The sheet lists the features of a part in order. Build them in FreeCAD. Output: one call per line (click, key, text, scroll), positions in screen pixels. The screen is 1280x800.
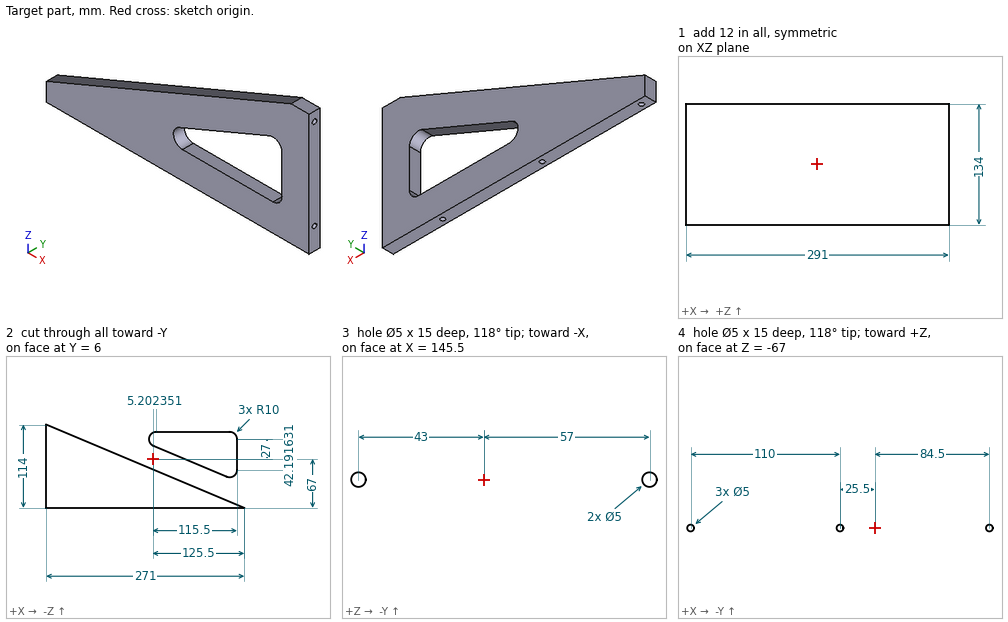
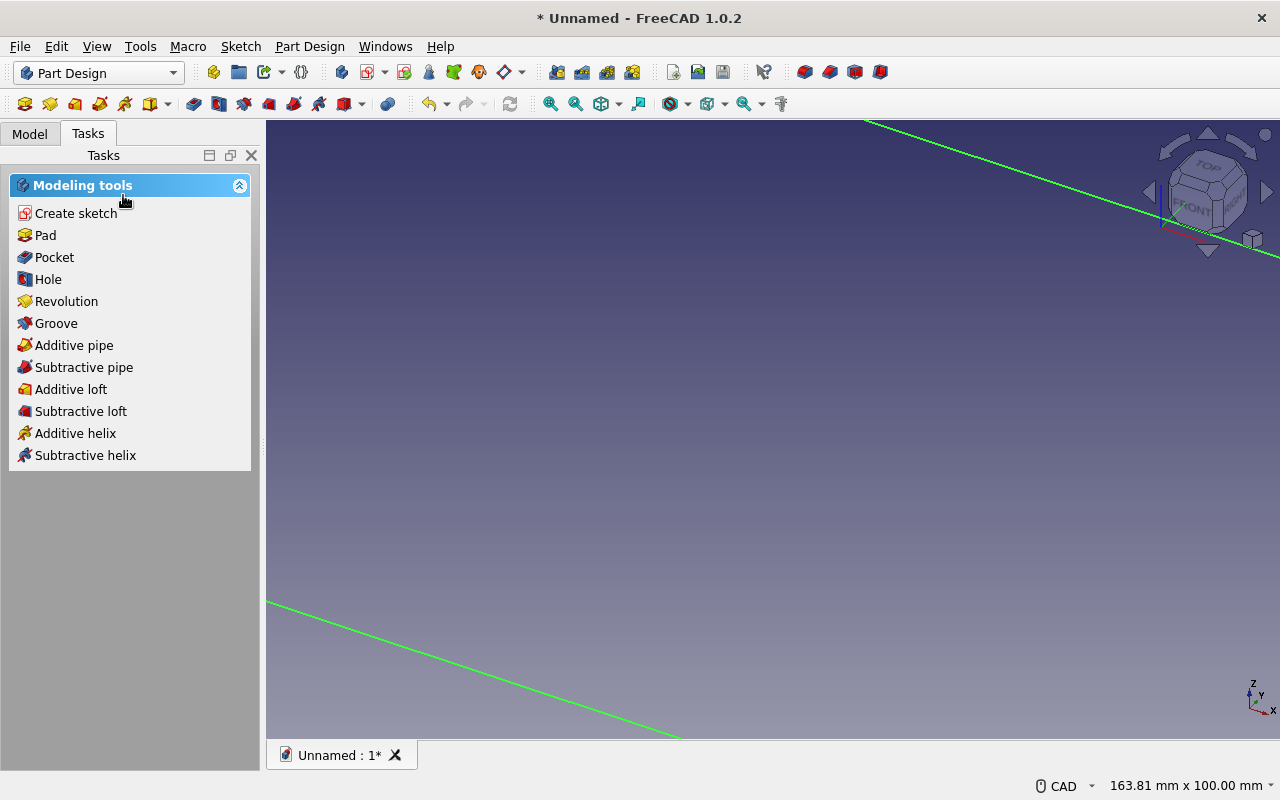
click(25, 104)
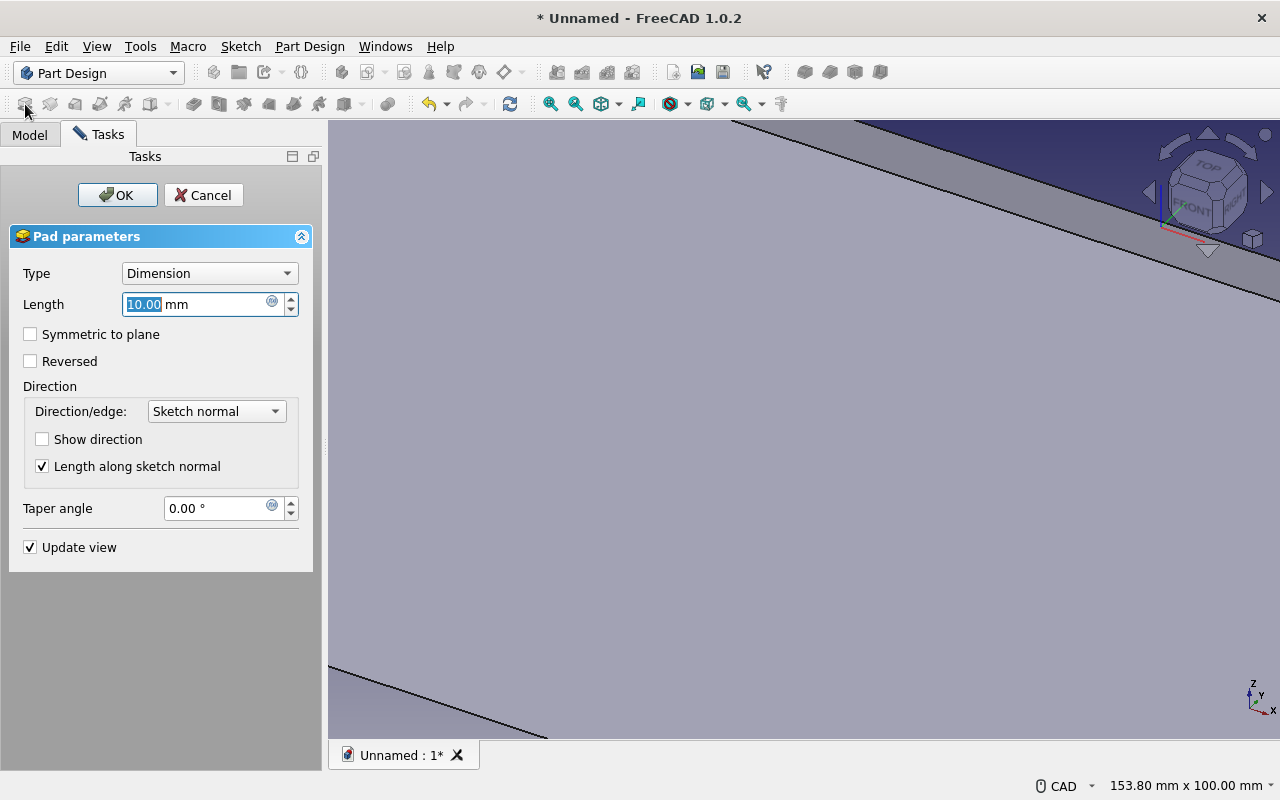
text(12)
key(Tab)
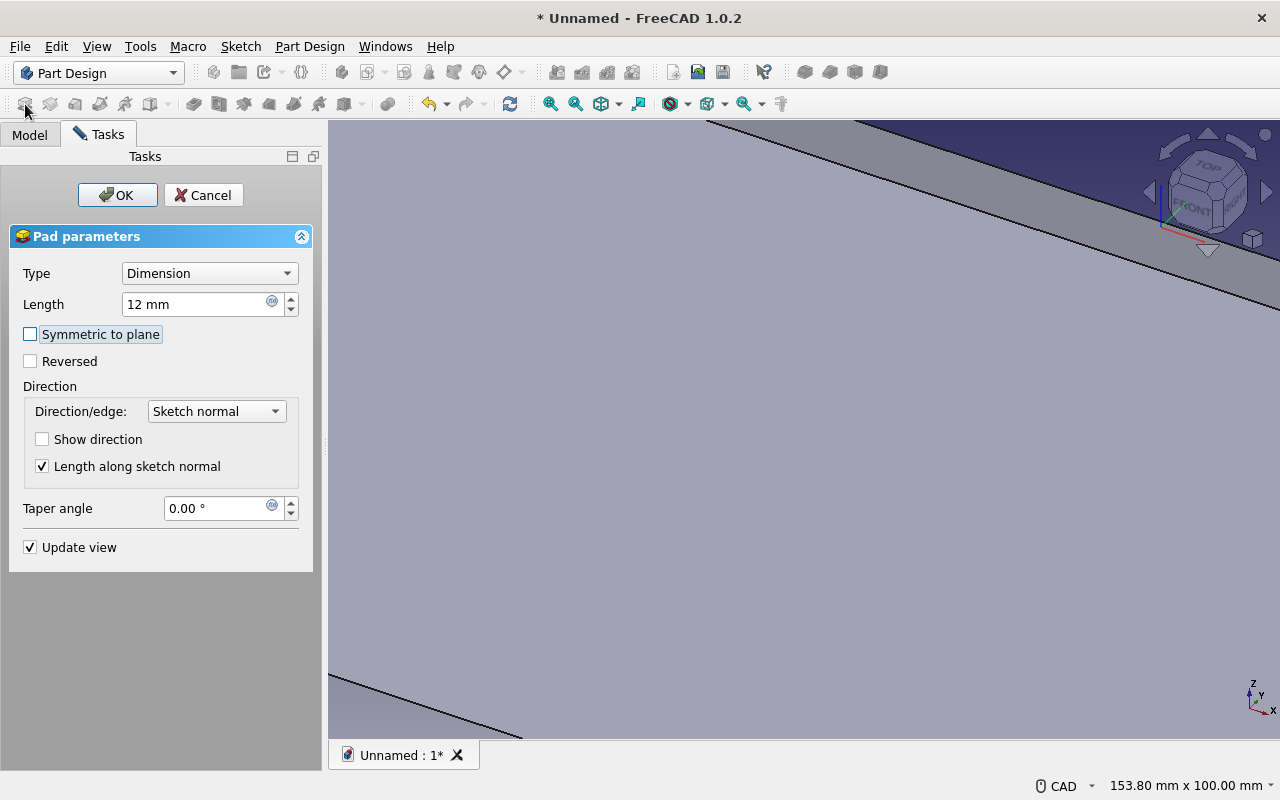
click(31, 334)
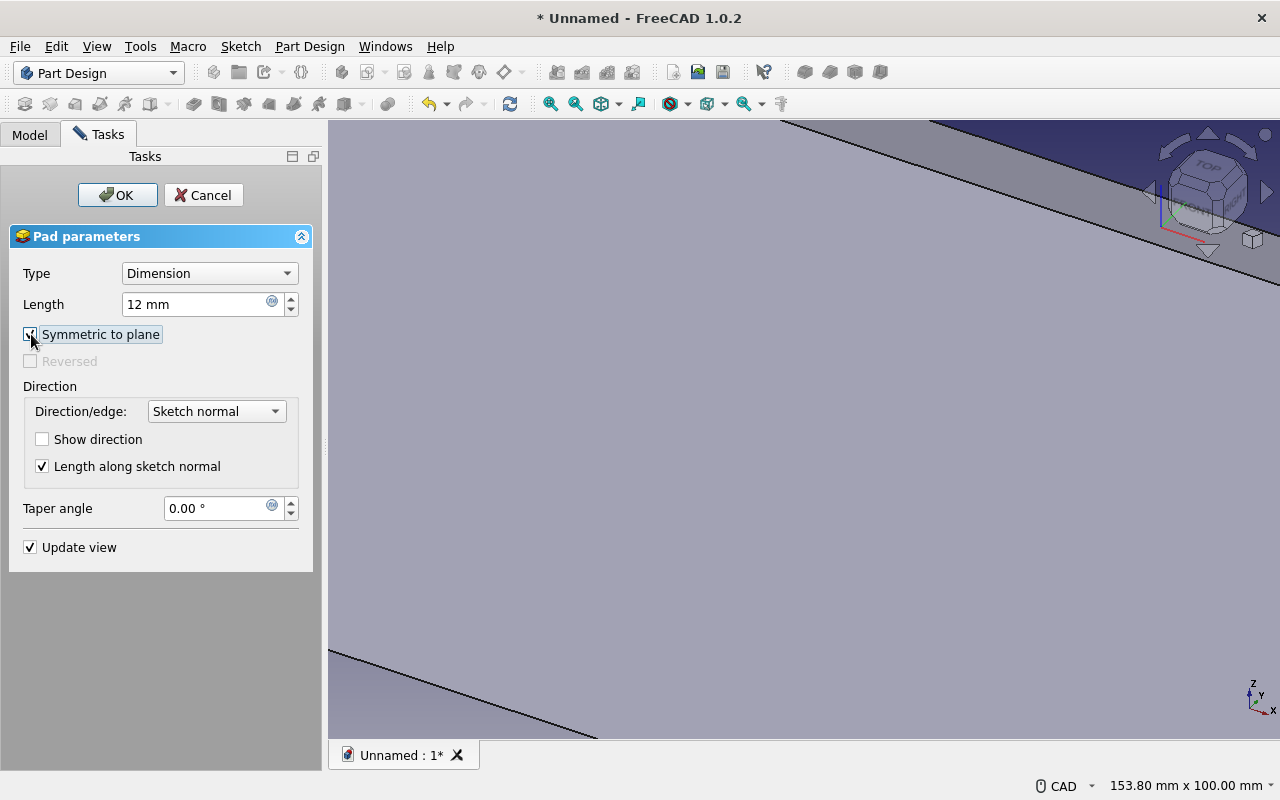
click(118, 195)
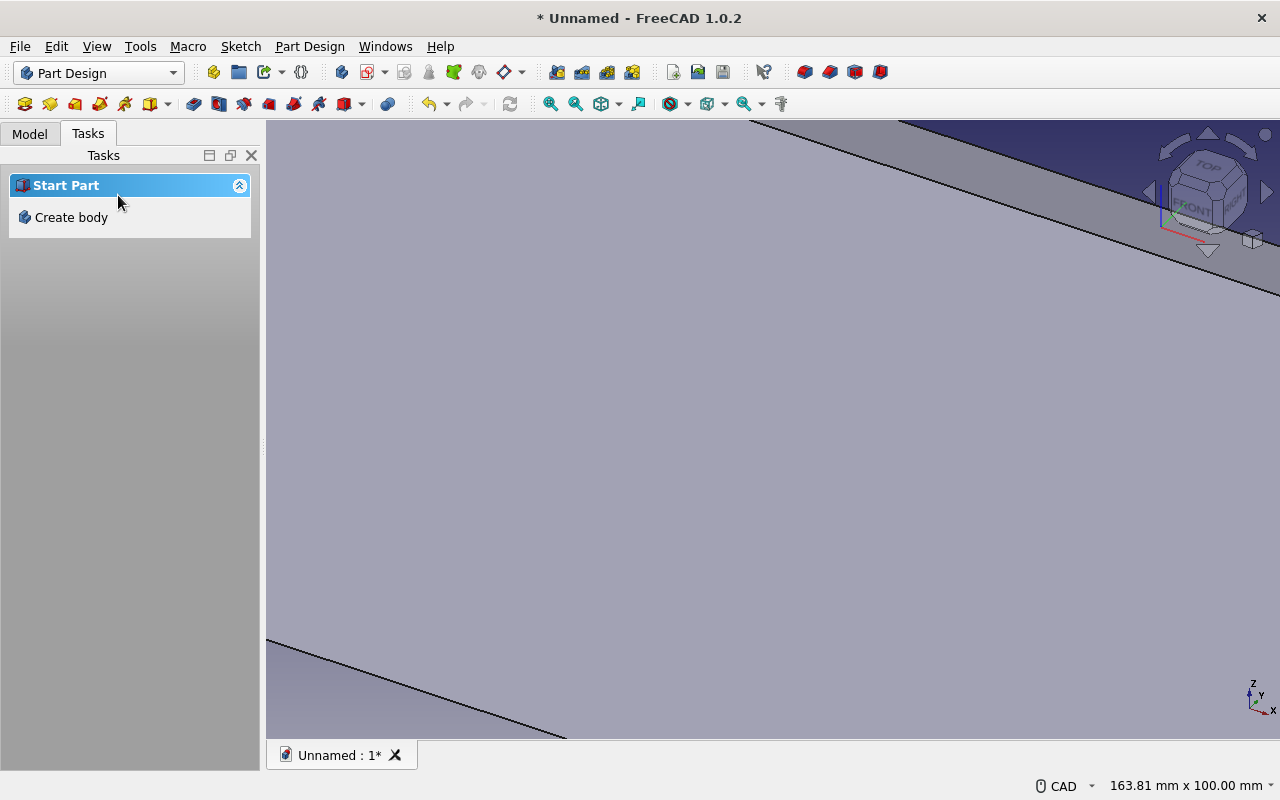
click(551, 104)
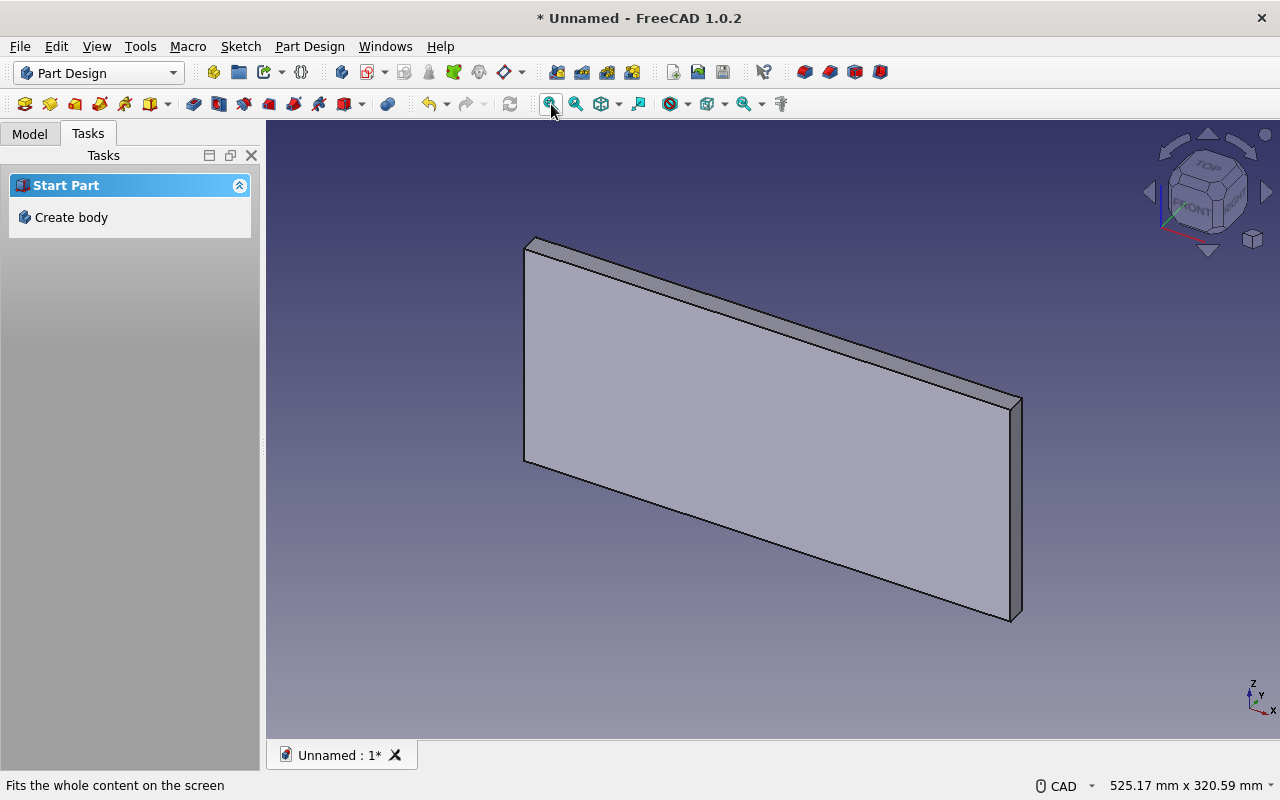
key(4)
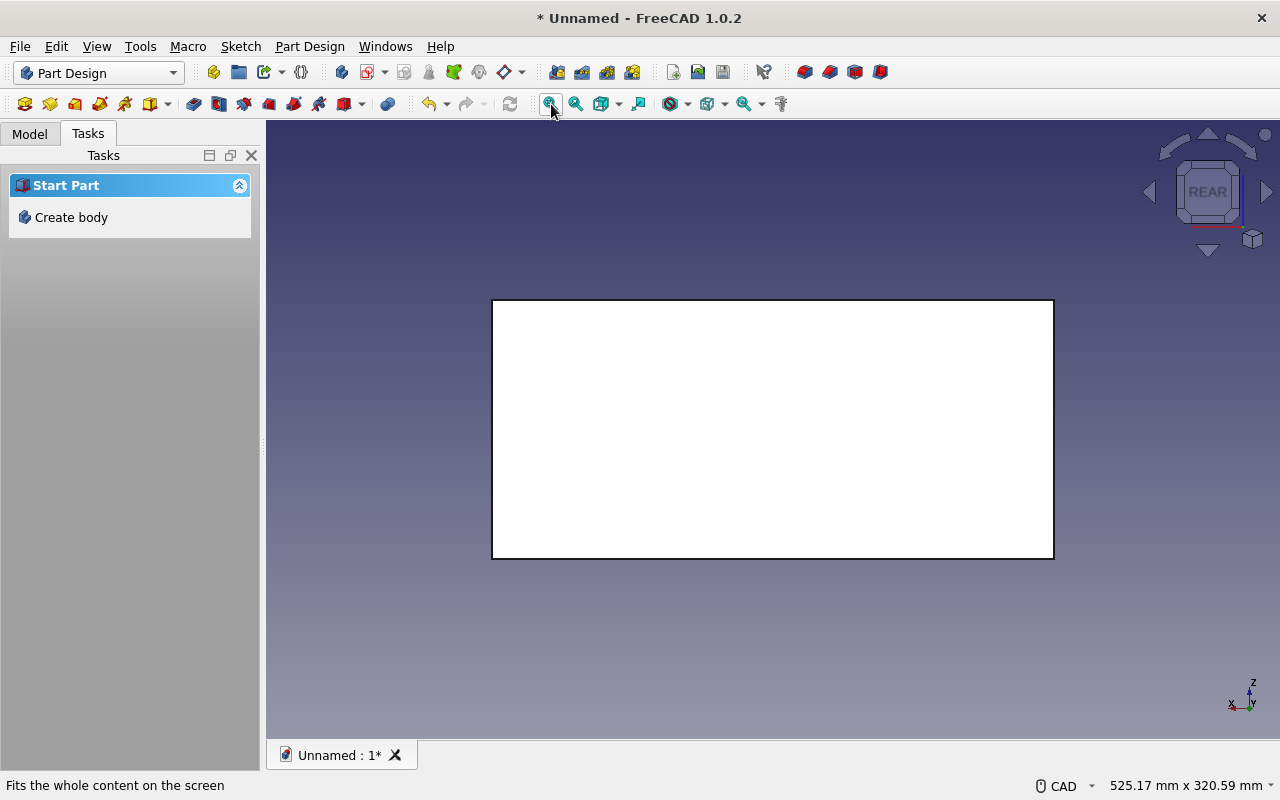
click(693, 429)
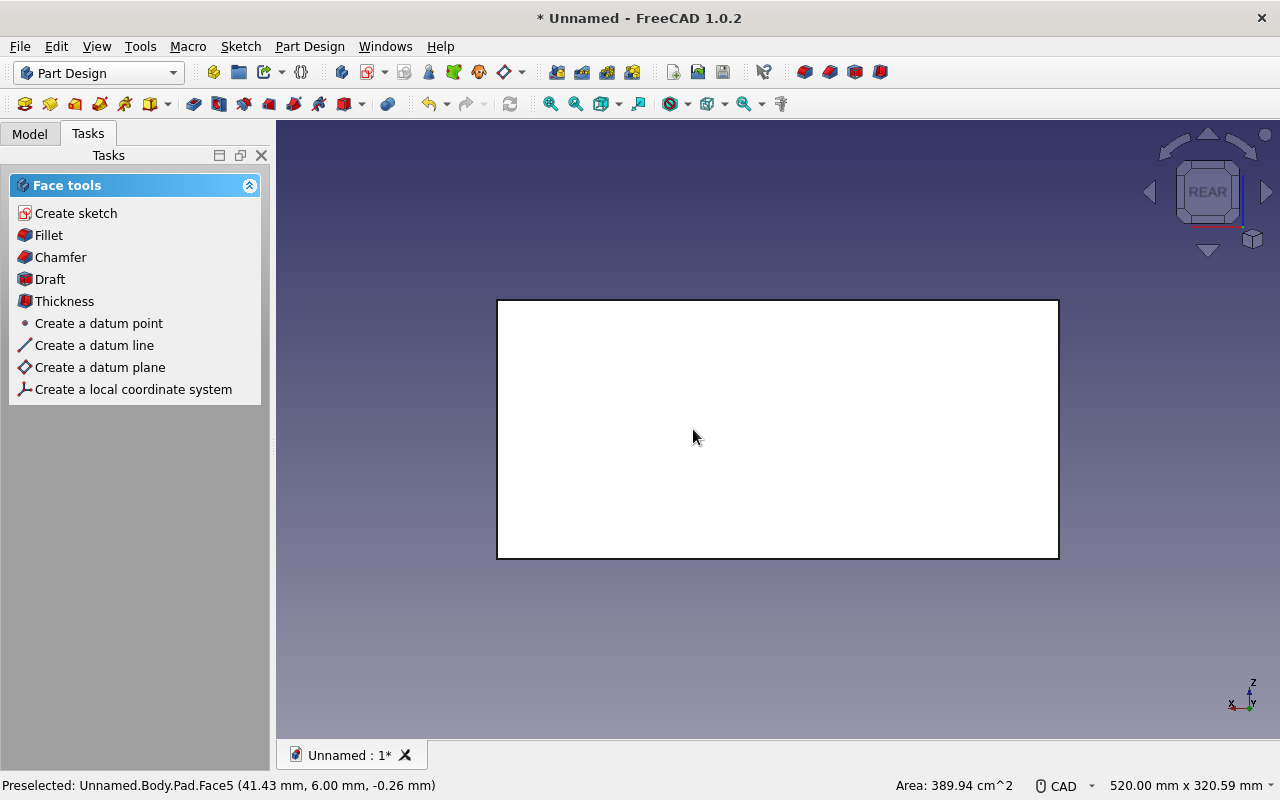
click(366, 72)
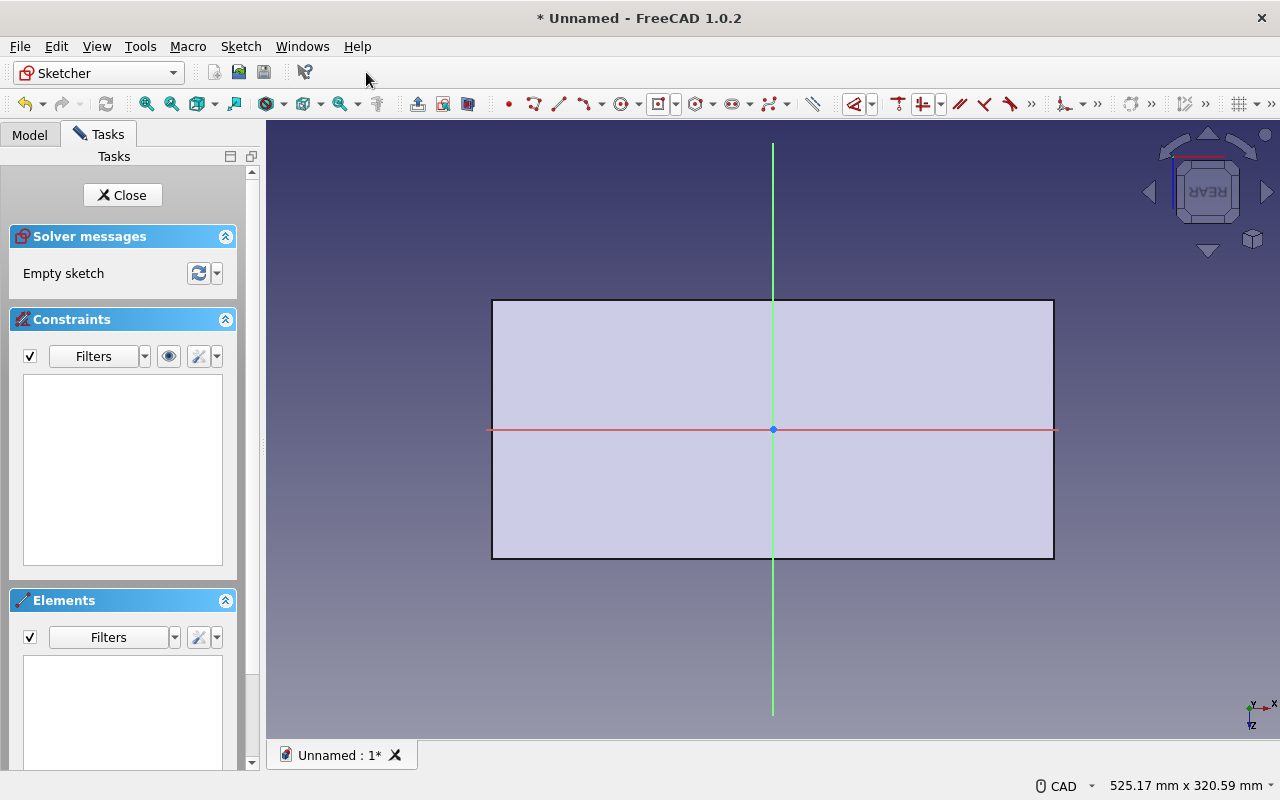
key(g)
key(m)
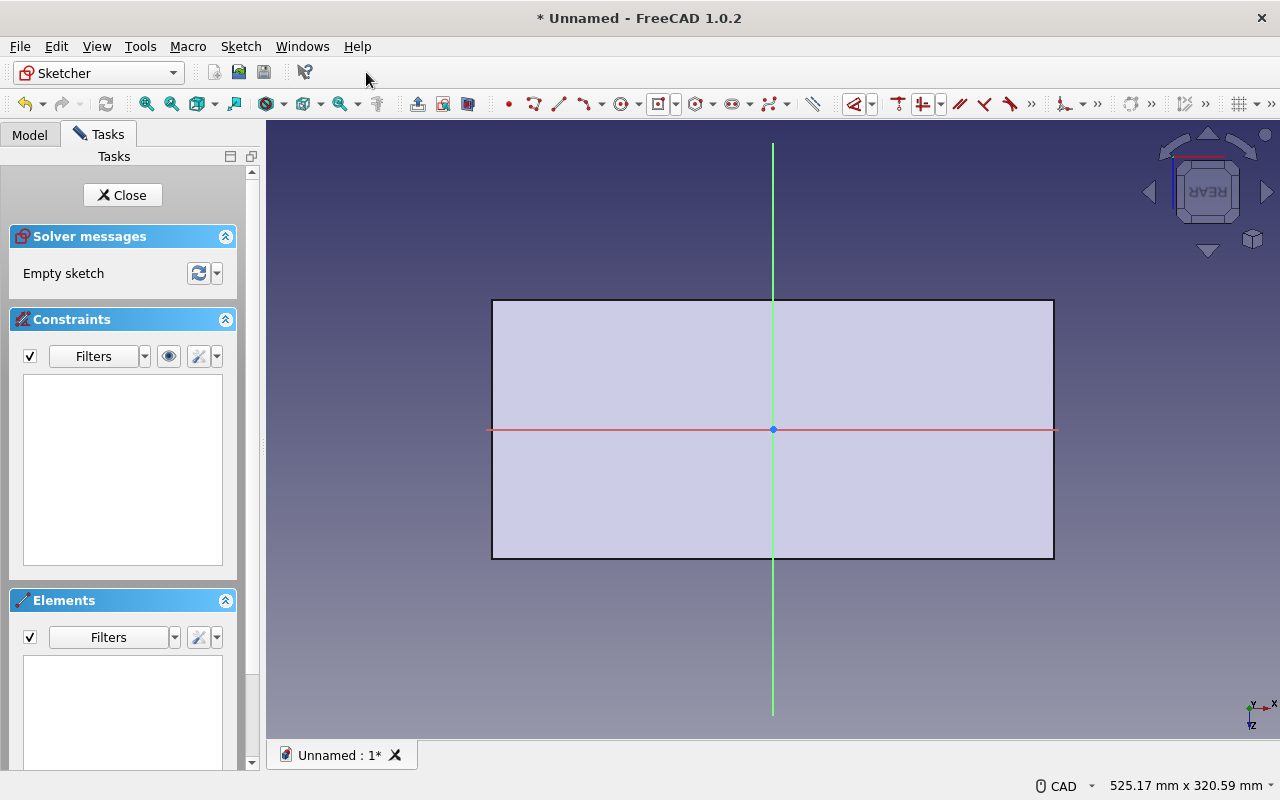
click(1015, 559)
click(492, 339)
click(492, 559)
click(1015, 560)